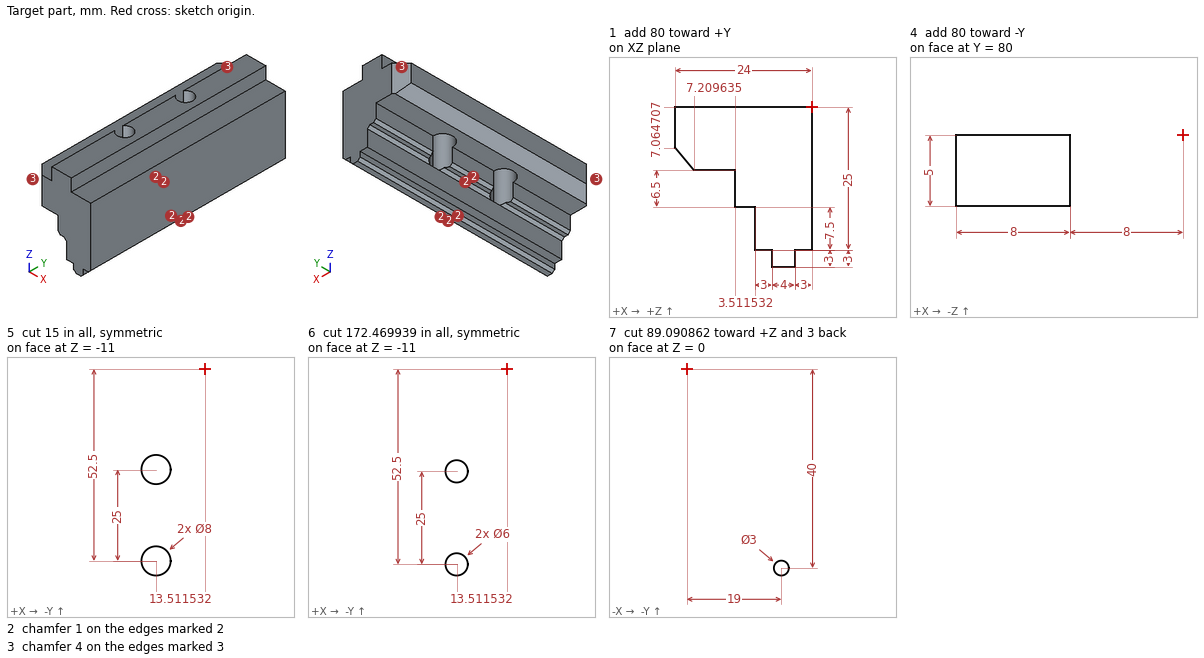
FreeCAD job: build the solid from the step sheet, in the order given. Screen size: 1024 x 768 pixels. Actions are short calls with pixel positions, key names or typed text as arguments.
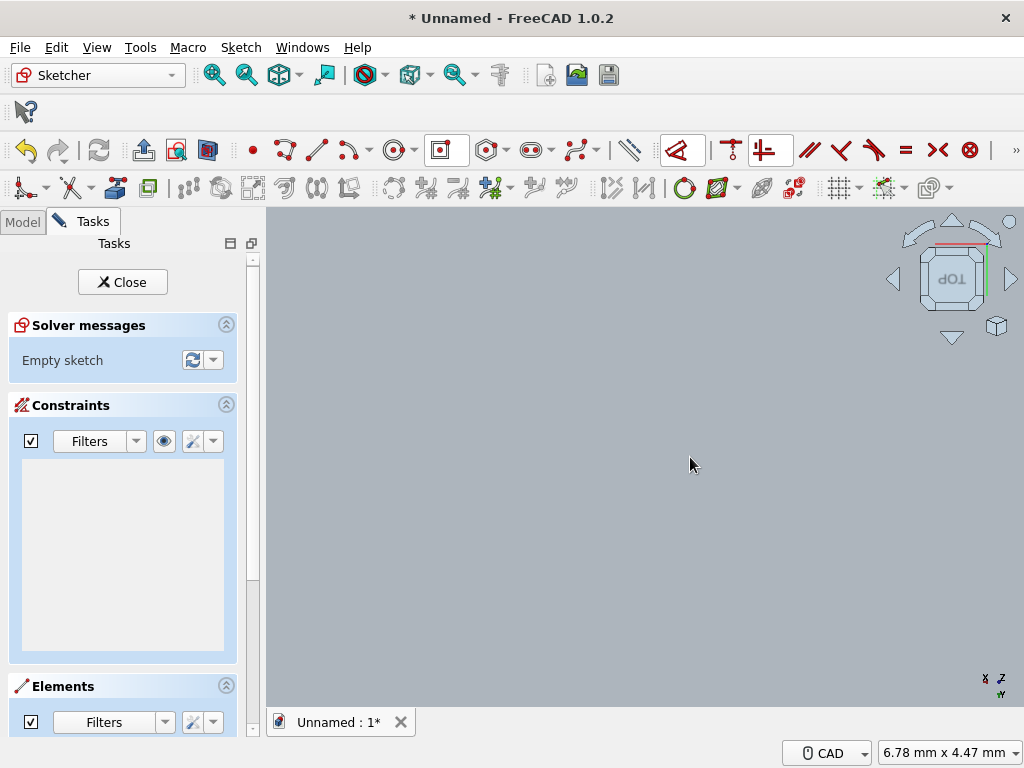
key(g)
key(c)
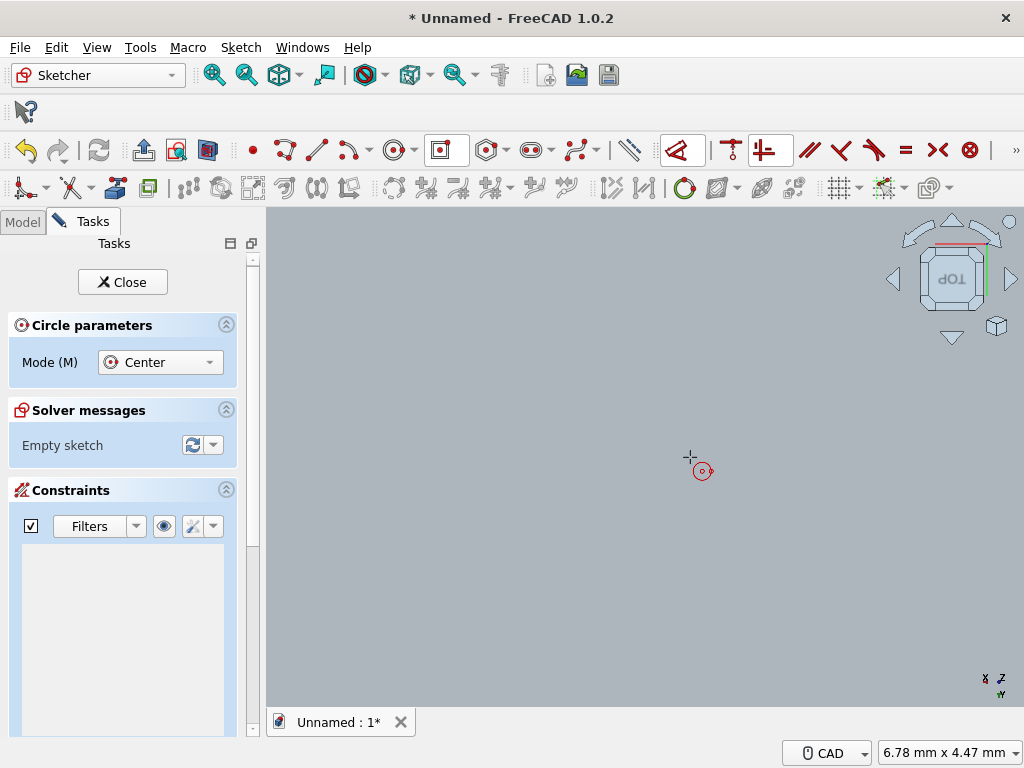
click(558, 447)
click(677, 329)
key(Escape)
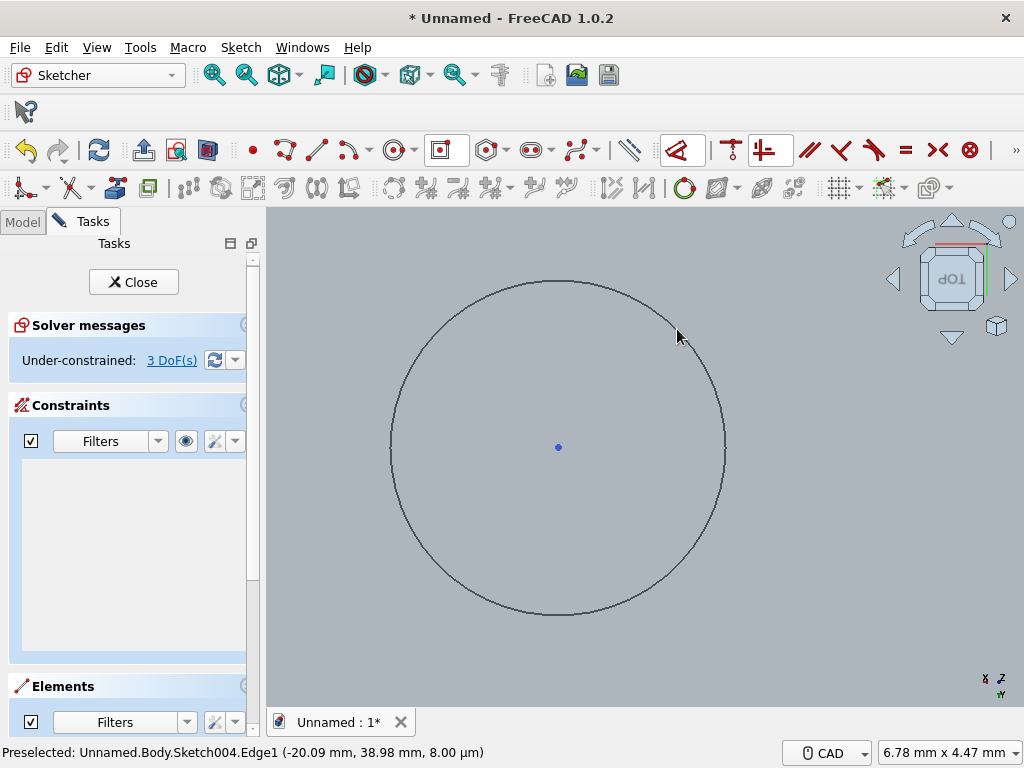
click(676, 329)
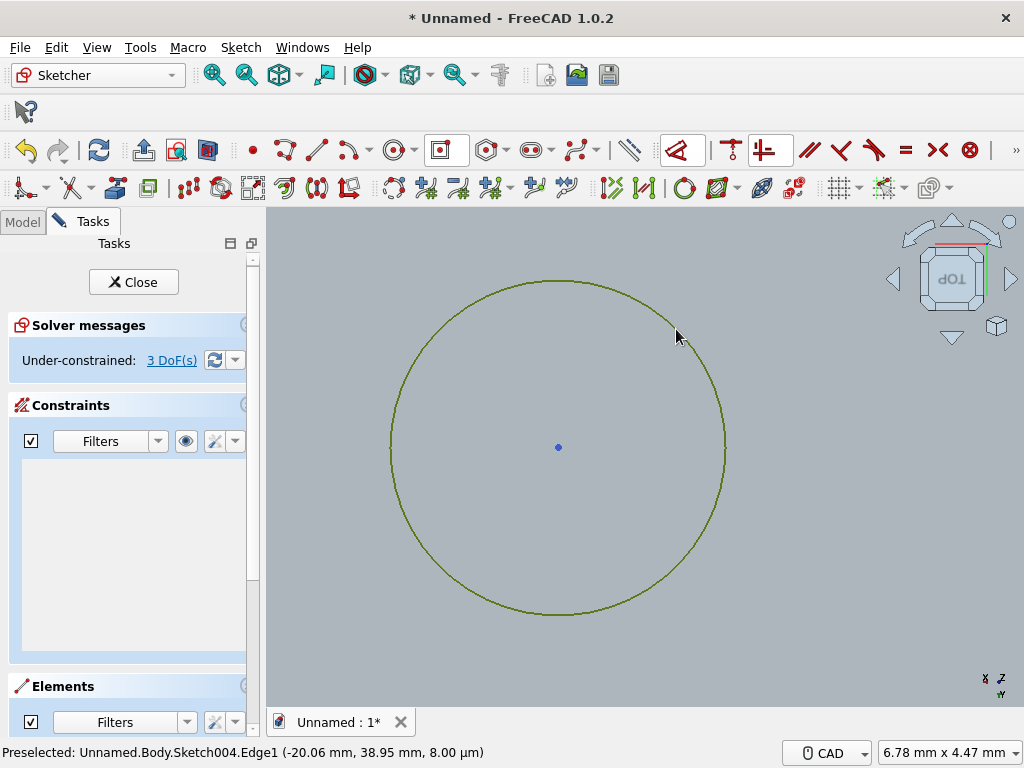
key(k)
key(o)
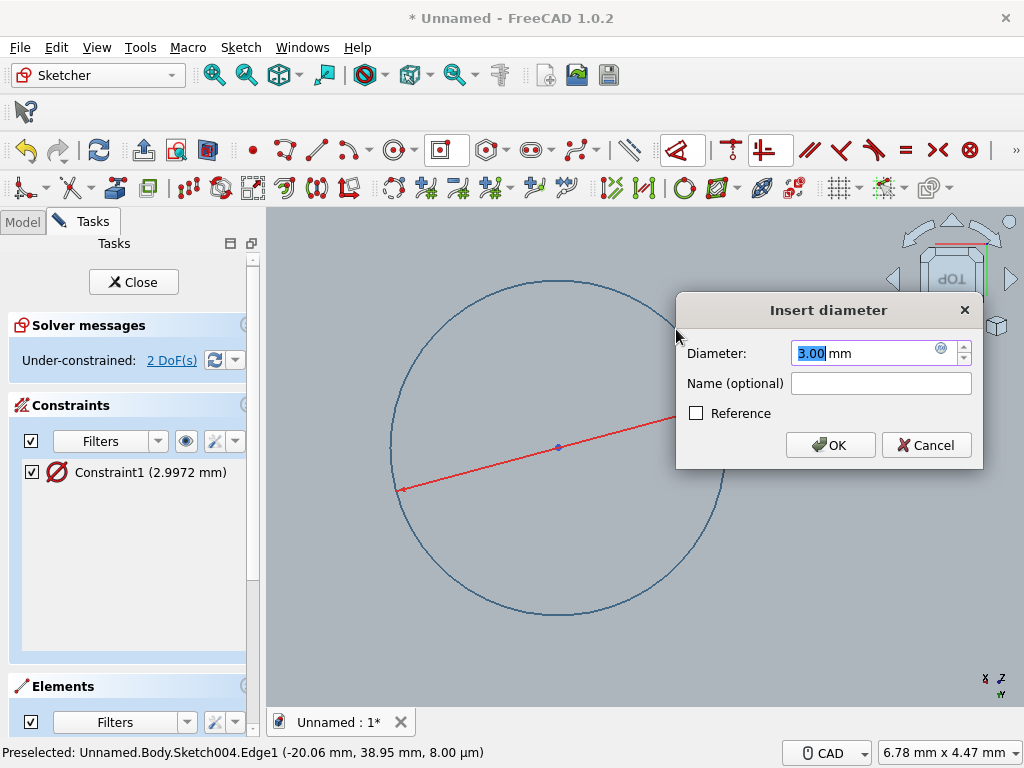
text(3)
key(Return)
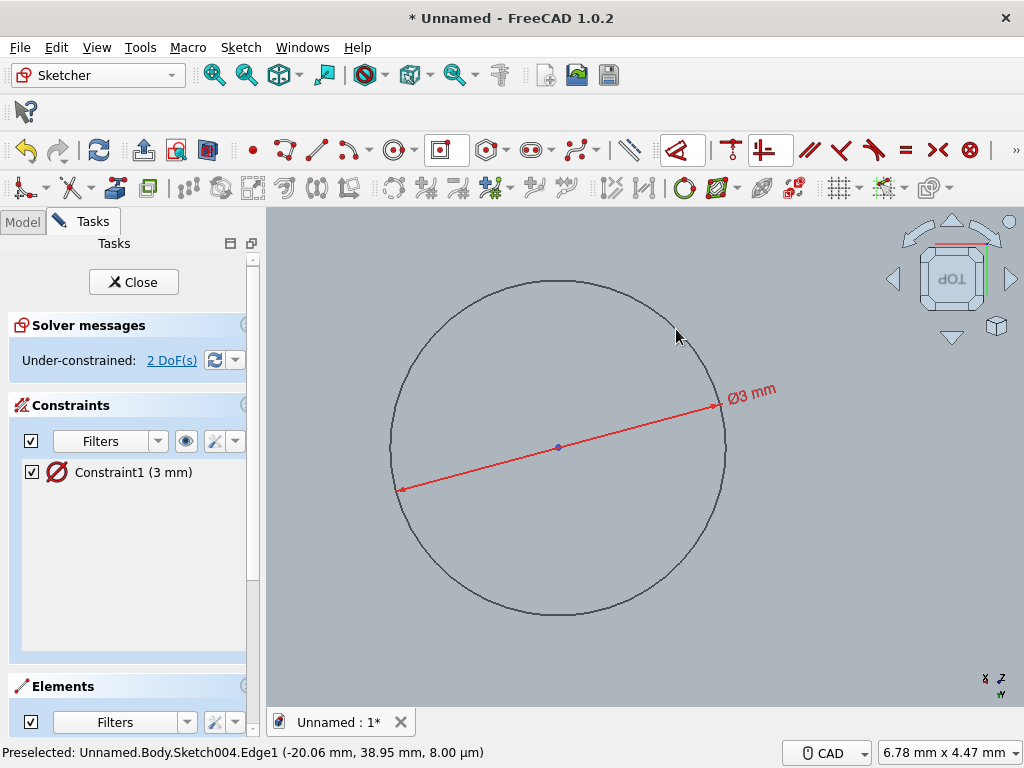
click(558, 448)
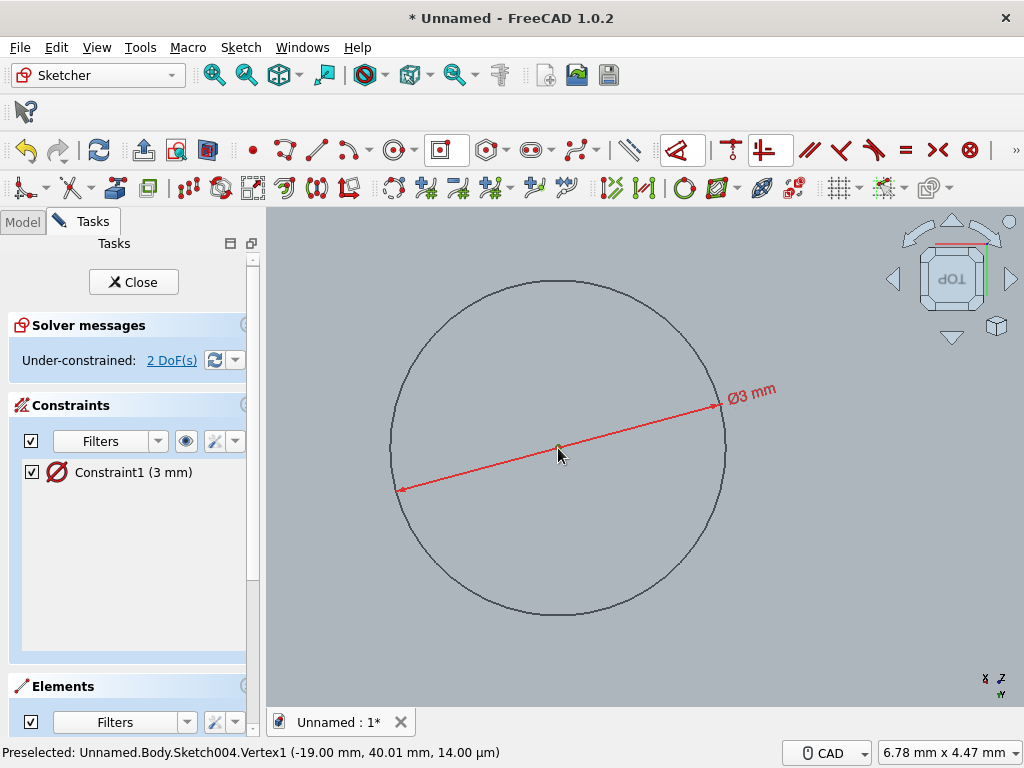
key(l)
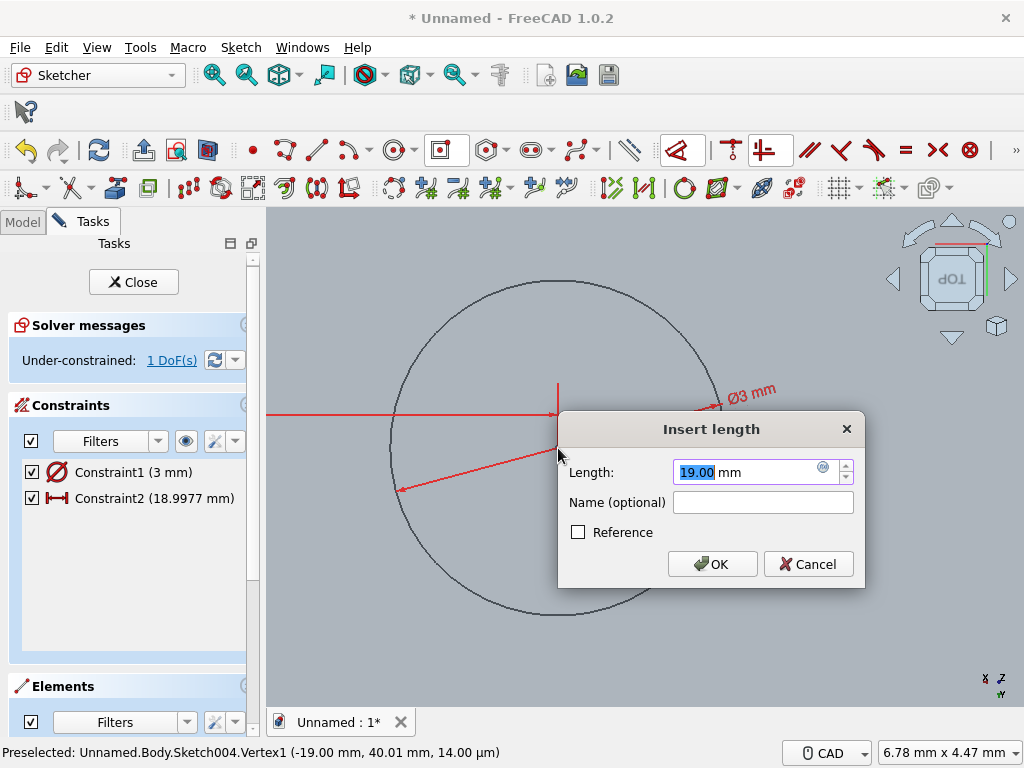
text(19)
key(Return)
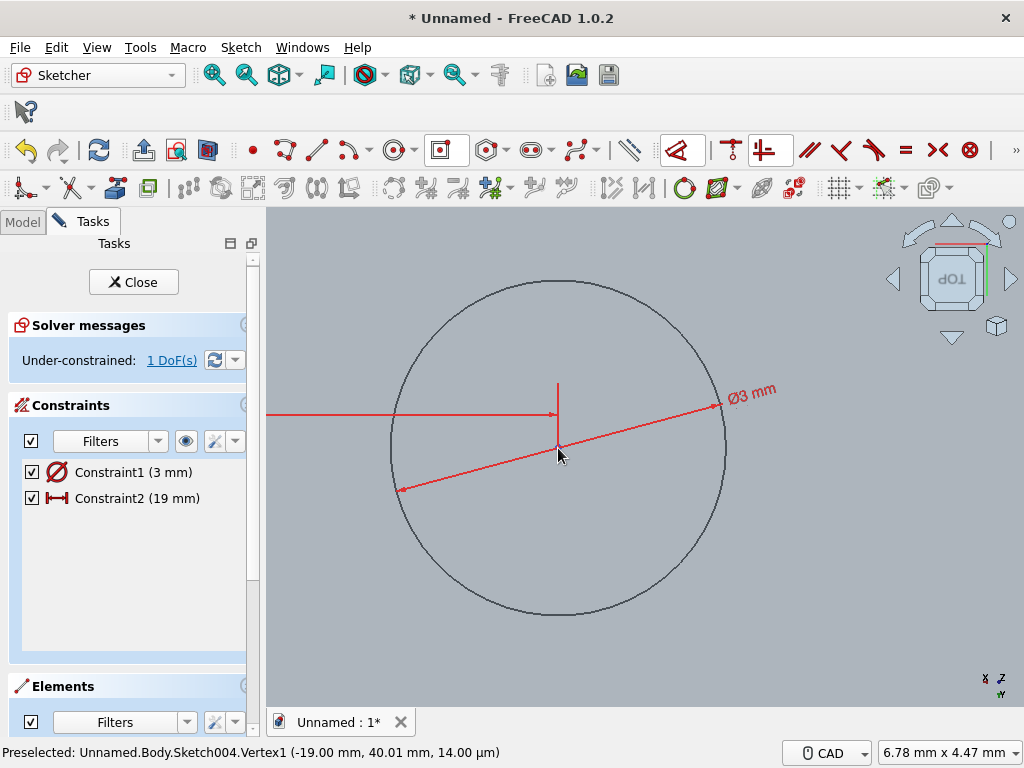
click(558, 448)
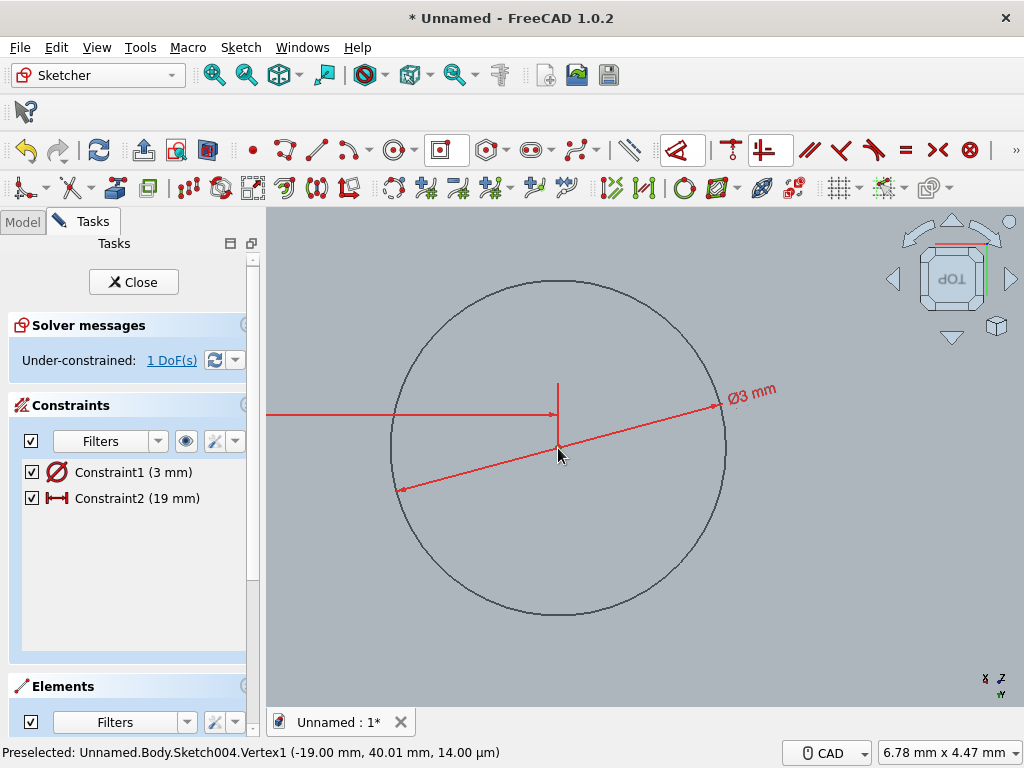
click(700, 150)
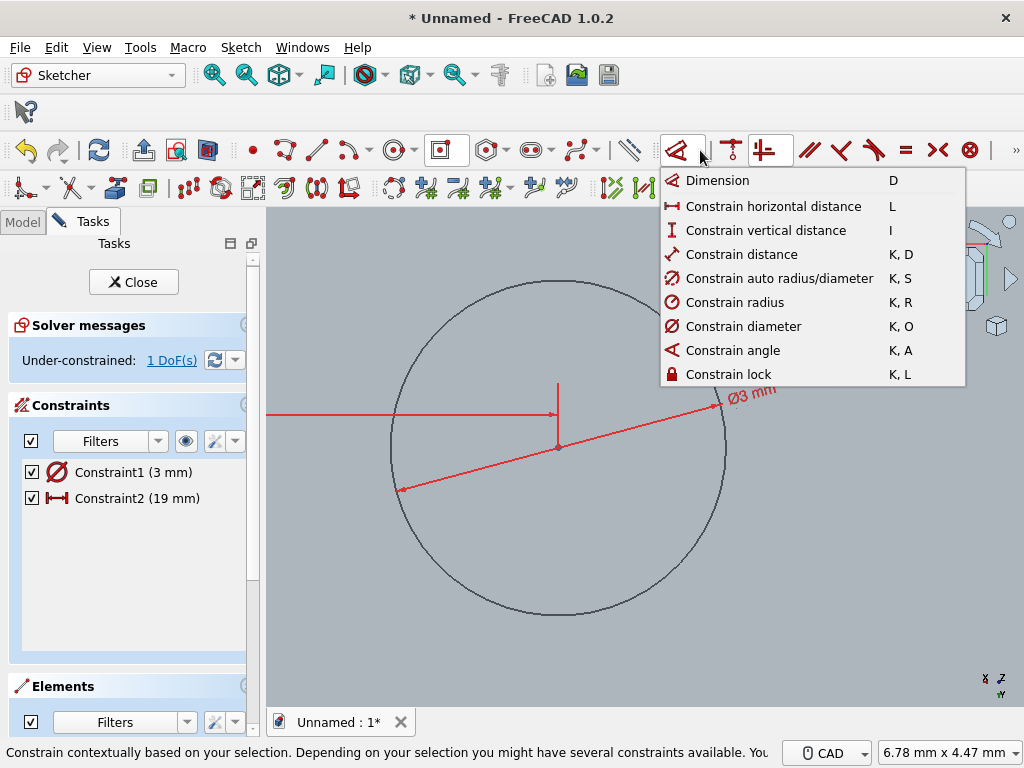
click(813, 230)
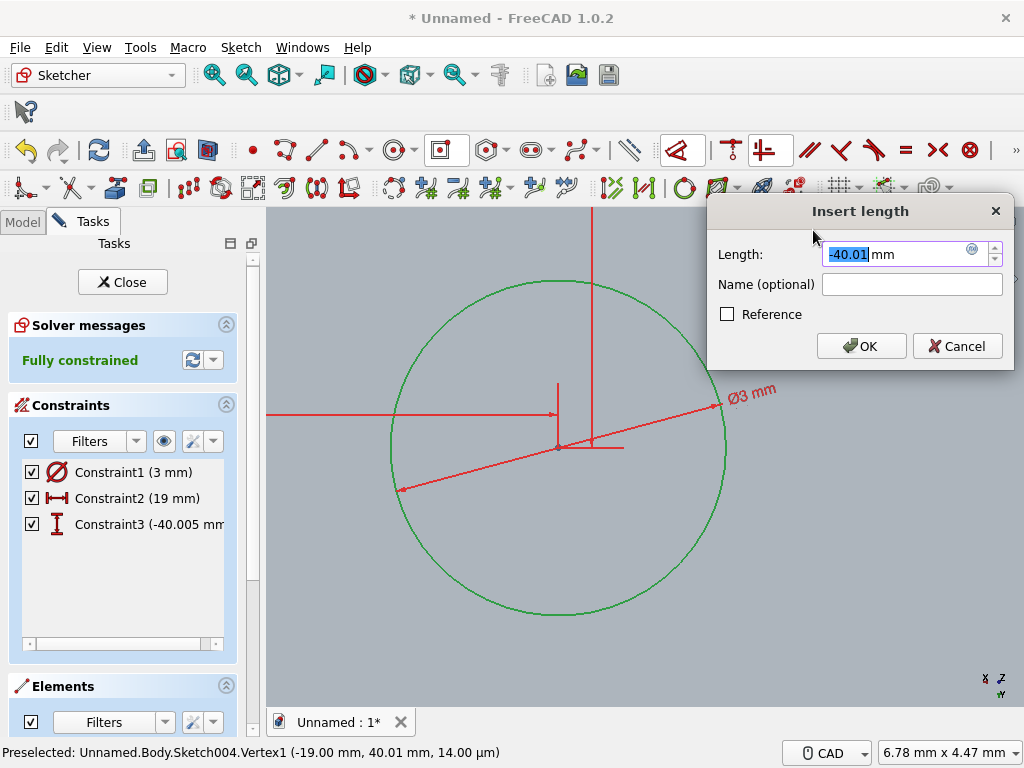
text(-40)
key(Return)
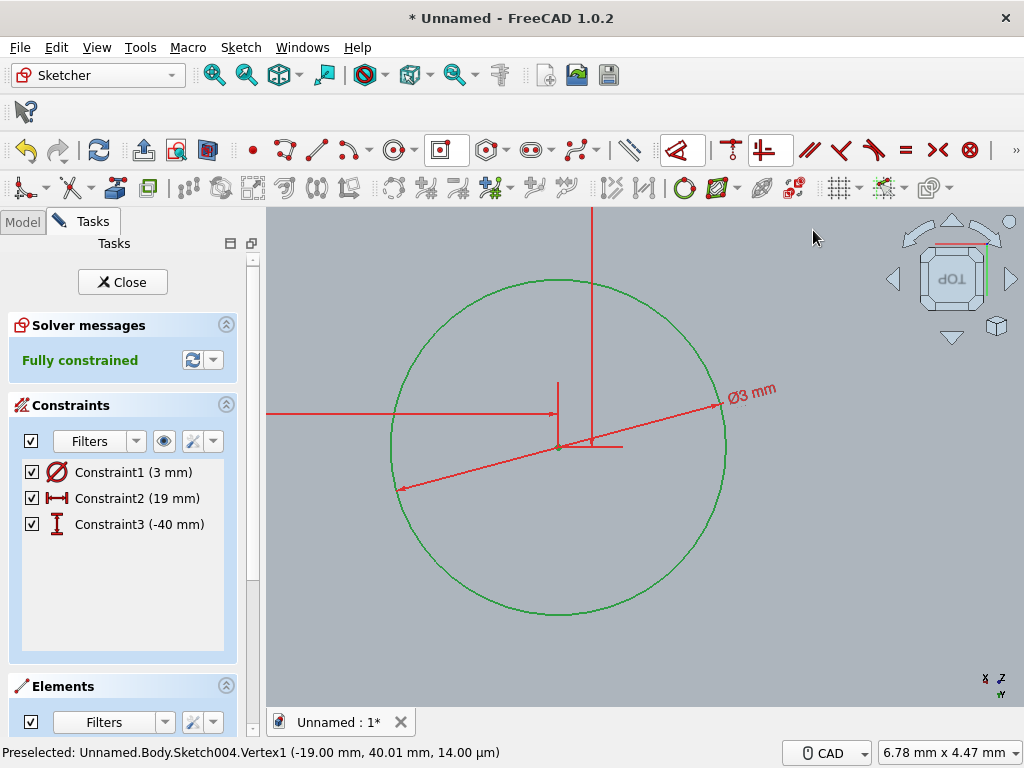
click(123, 282)